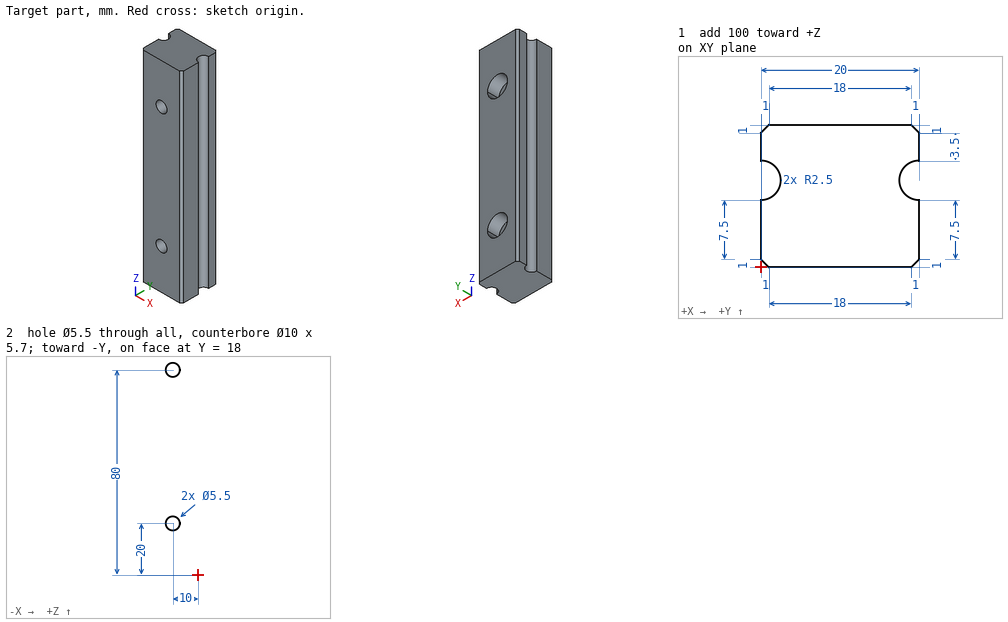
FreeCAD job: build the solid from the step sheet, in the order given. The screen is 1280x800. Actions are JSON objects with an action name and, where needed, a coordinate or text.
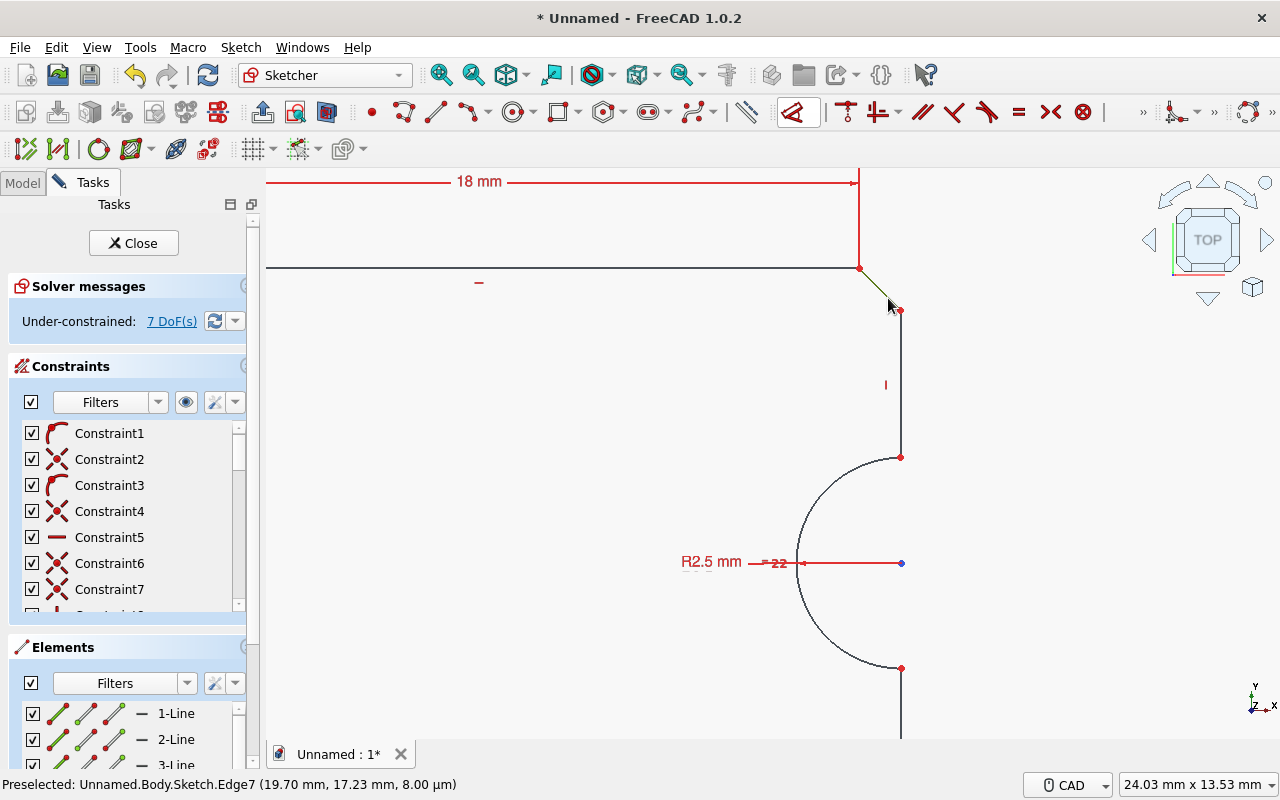
{"action": "key", "text": "l"}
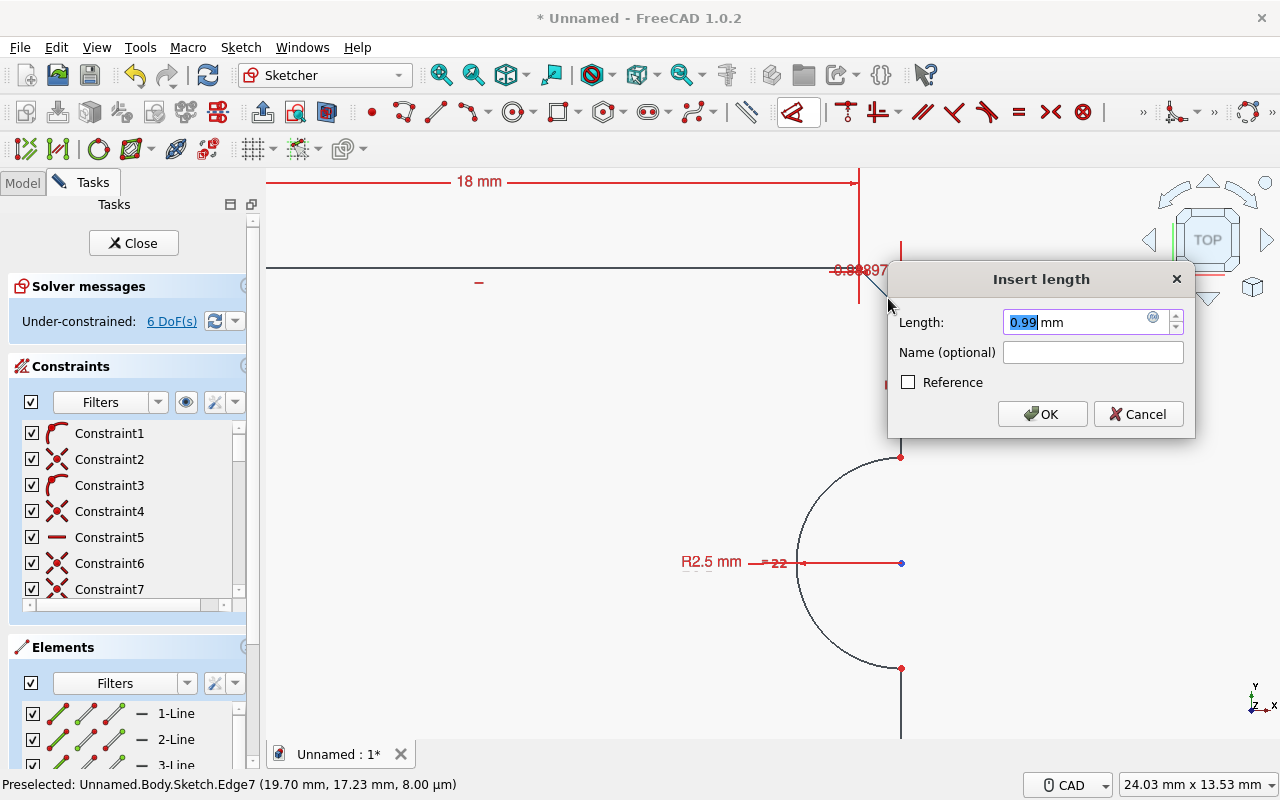
{"action": "type", "text": "1"}
{"action": "key", "text": "Return"}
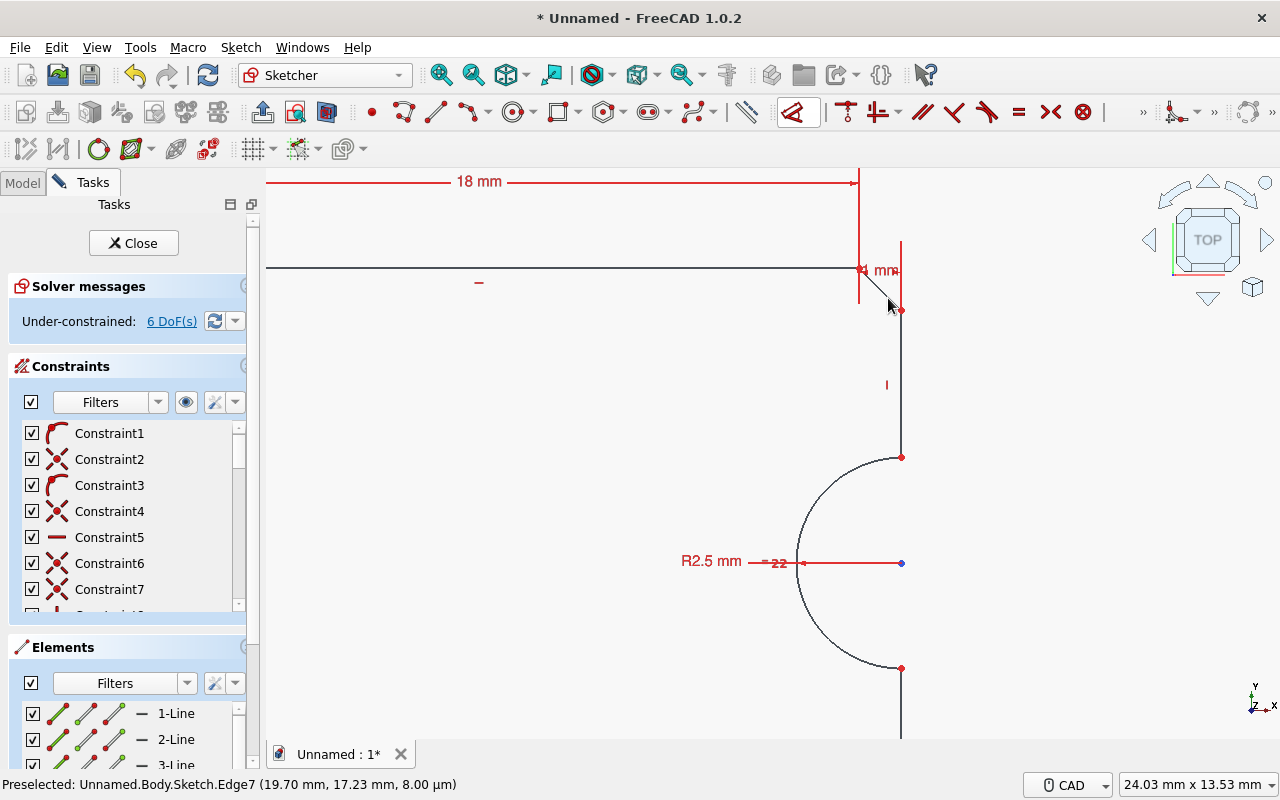
{"action": "left_click", "coordinate": [889, 298]}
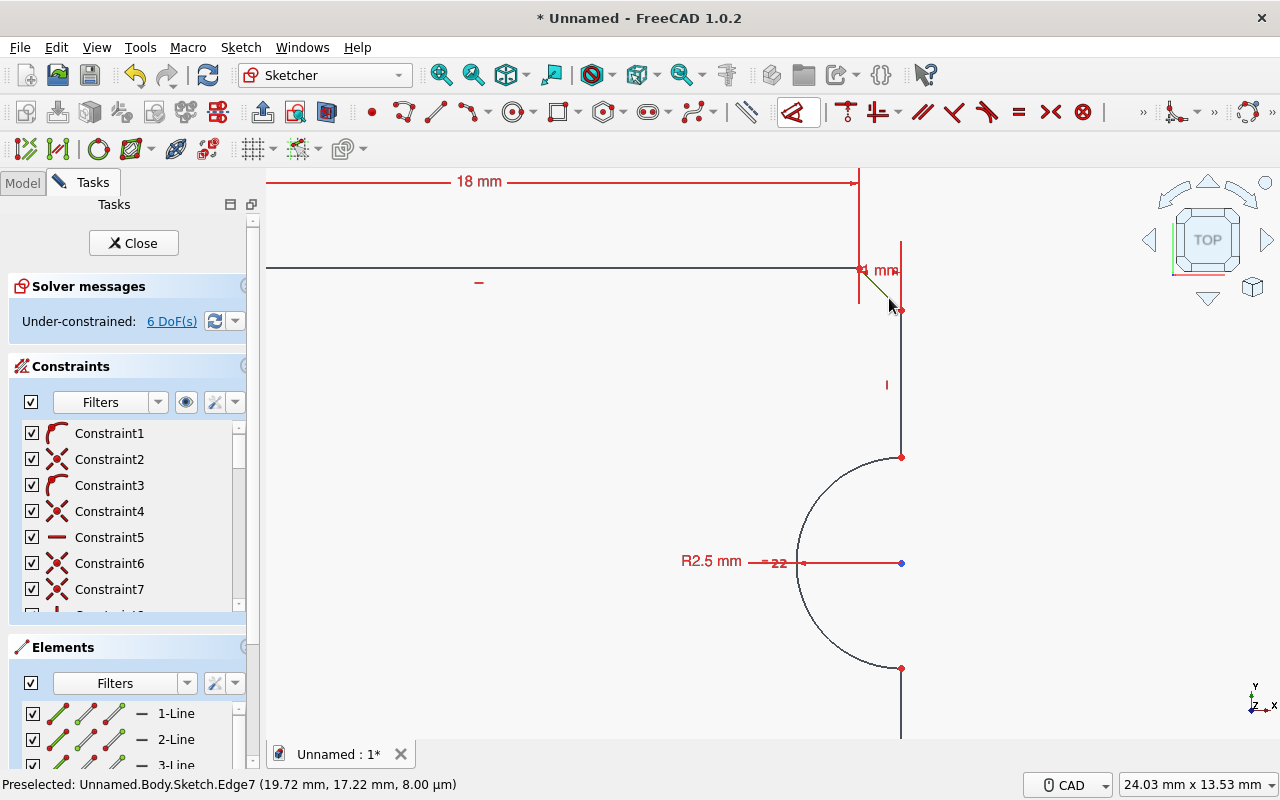
{"action": "left_click", "coordinate": [814, 112]}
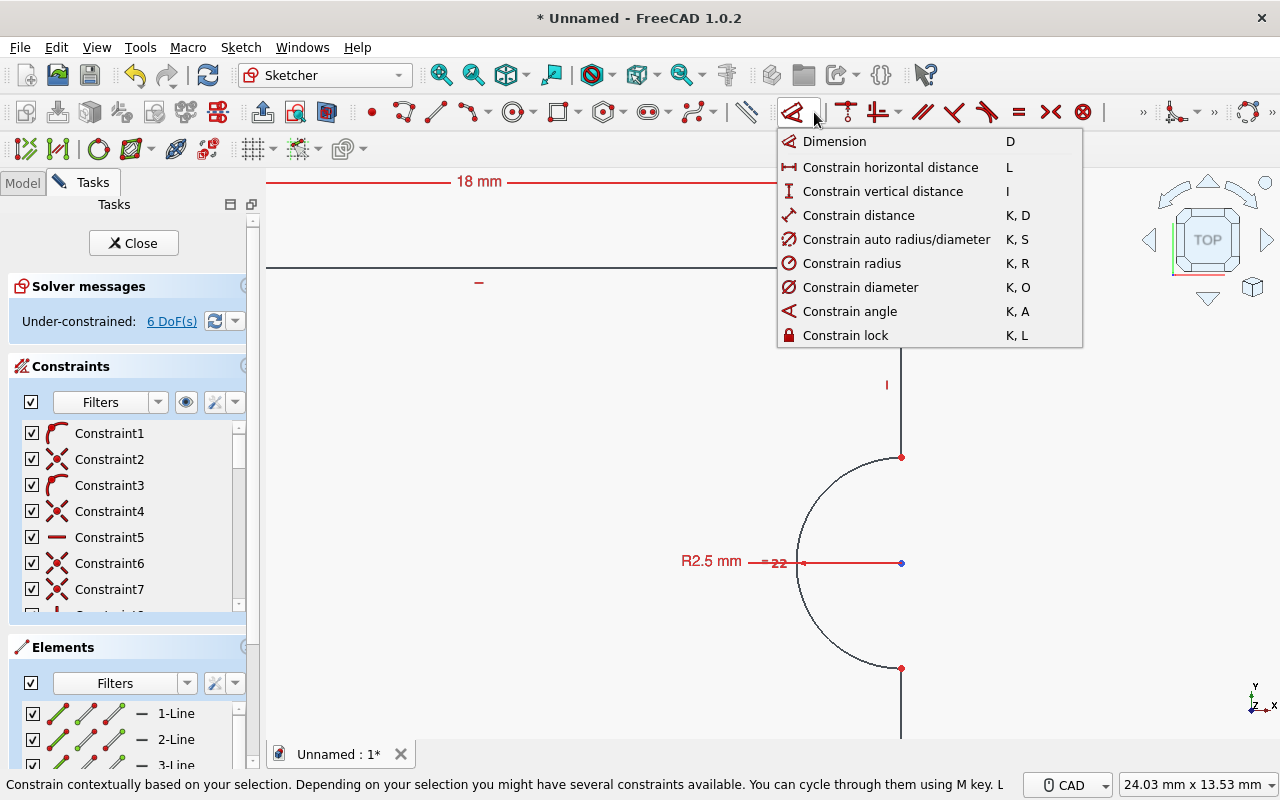
{"action": "left_click", "coordinate": [930, 191]}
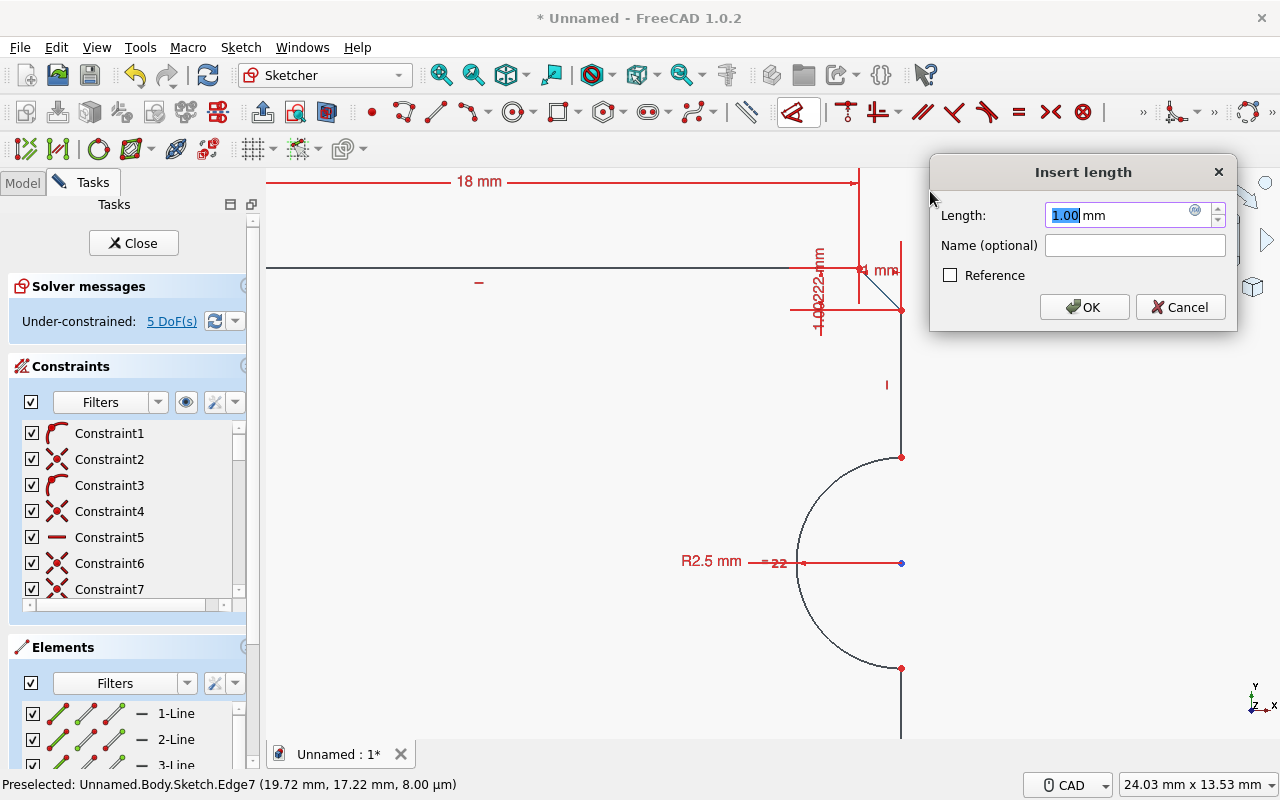
{"action": "type", "text": "1"}
{"action": "key", "text": "Return"}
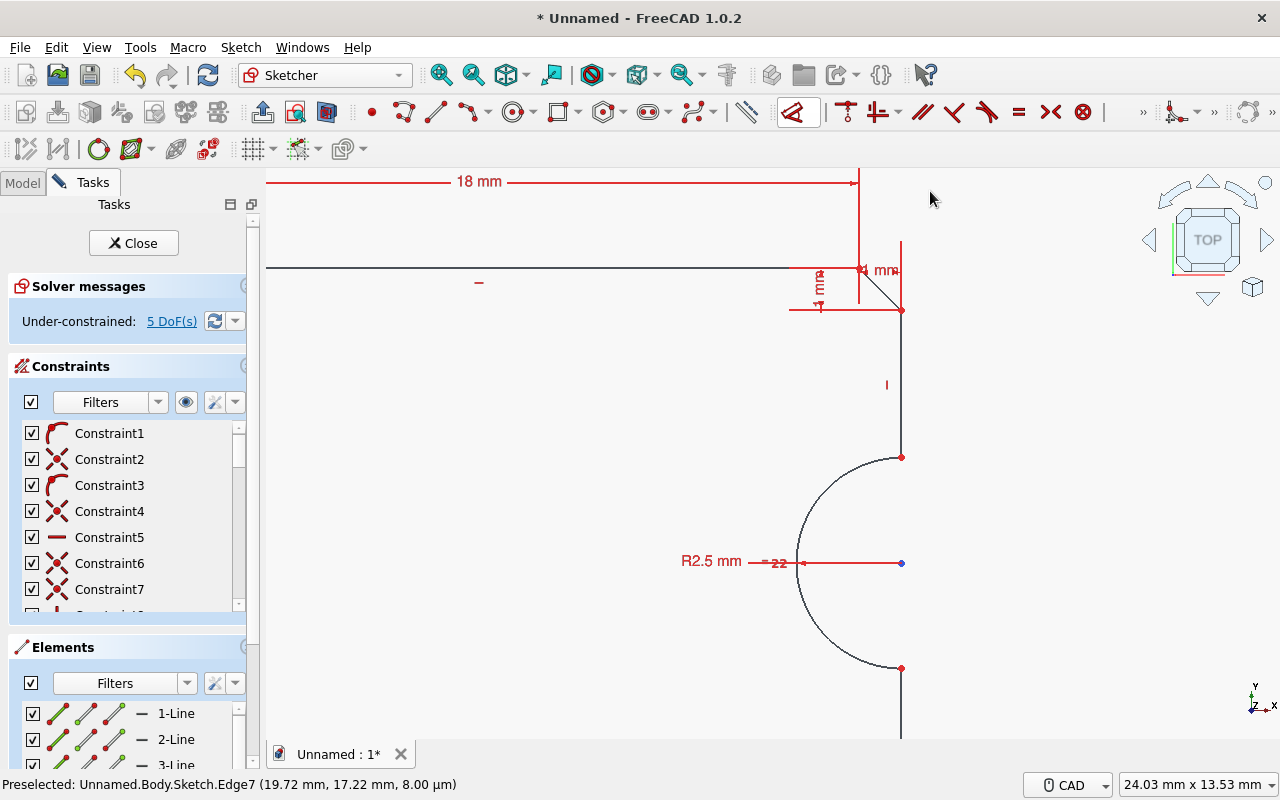
{"action": "scroll", "coordinate": [888, 297], "scroll_direction": "down", "scroll_amount": 4}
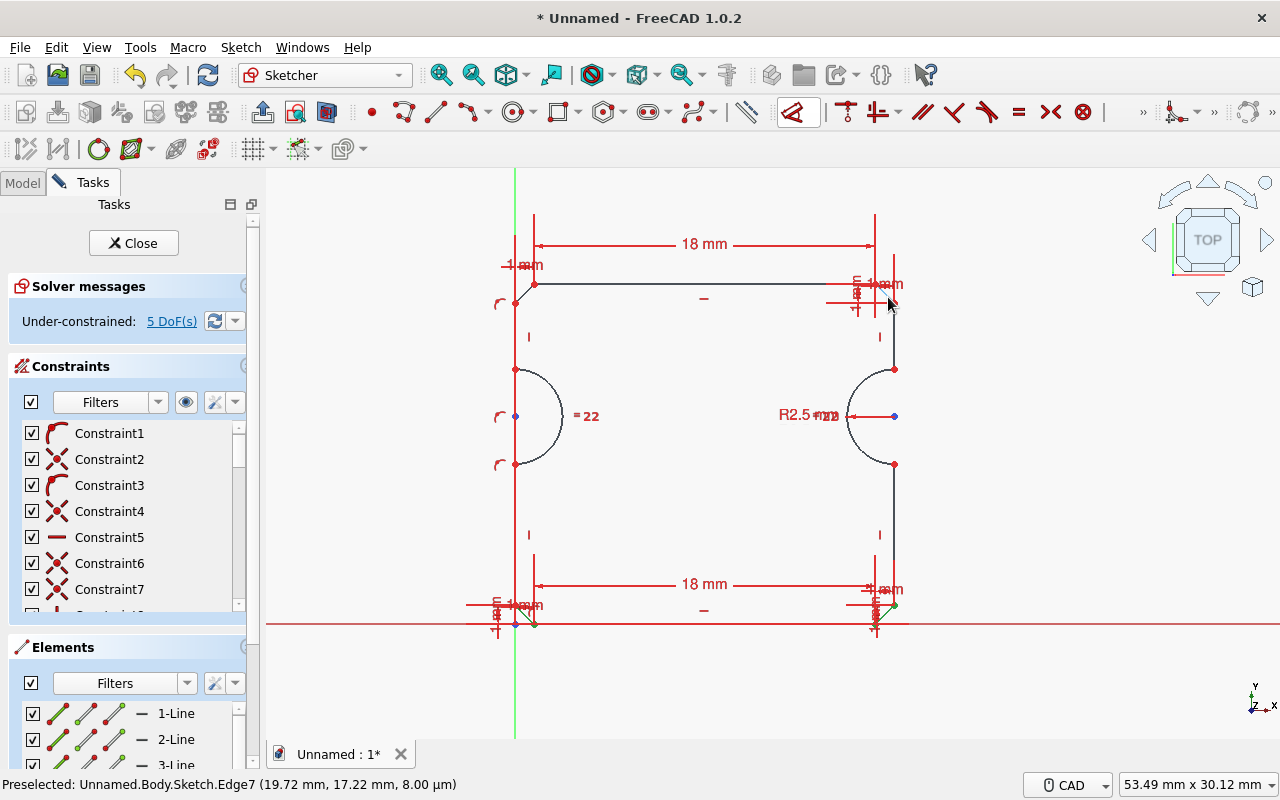
{"action": "scroll", "coordinate": [528, 290], "scroll_direction": "up", "scroll_amount": 4}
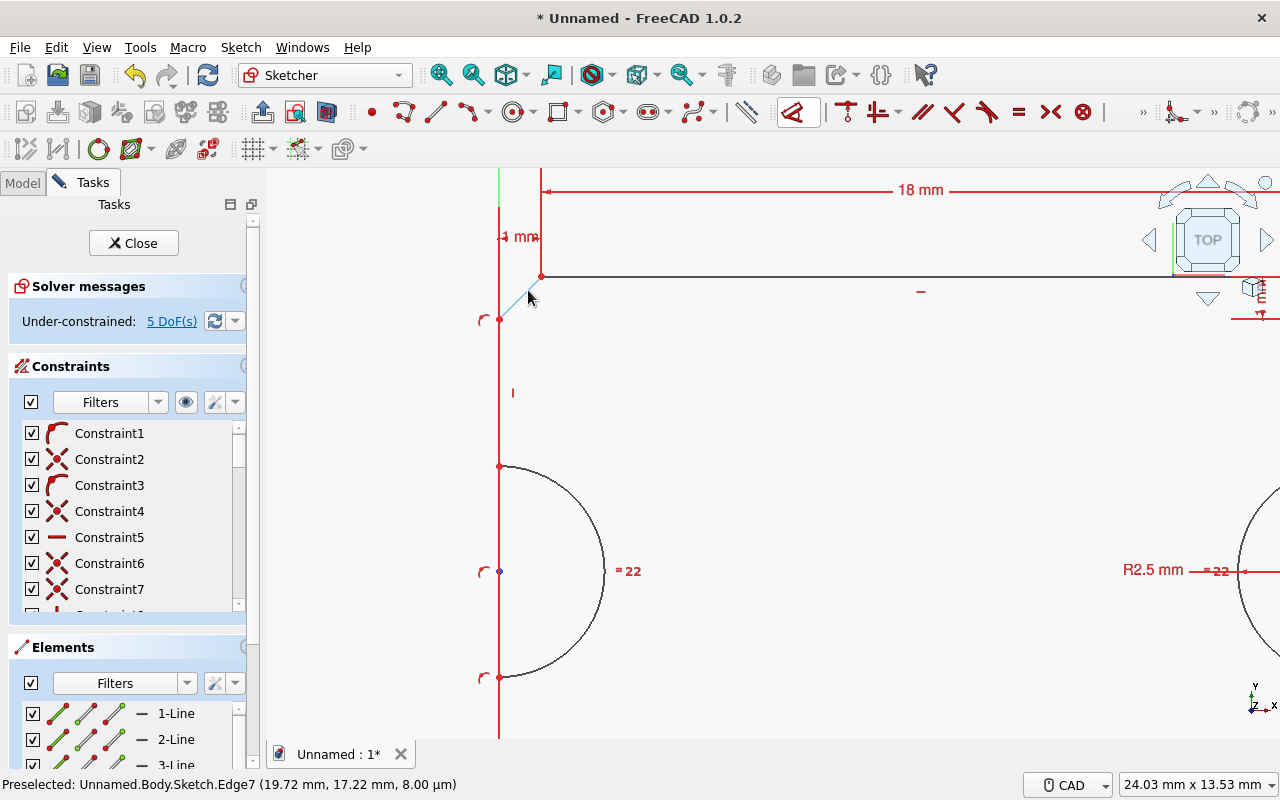
{"action": "left_click", "coordinate": [529, 289]}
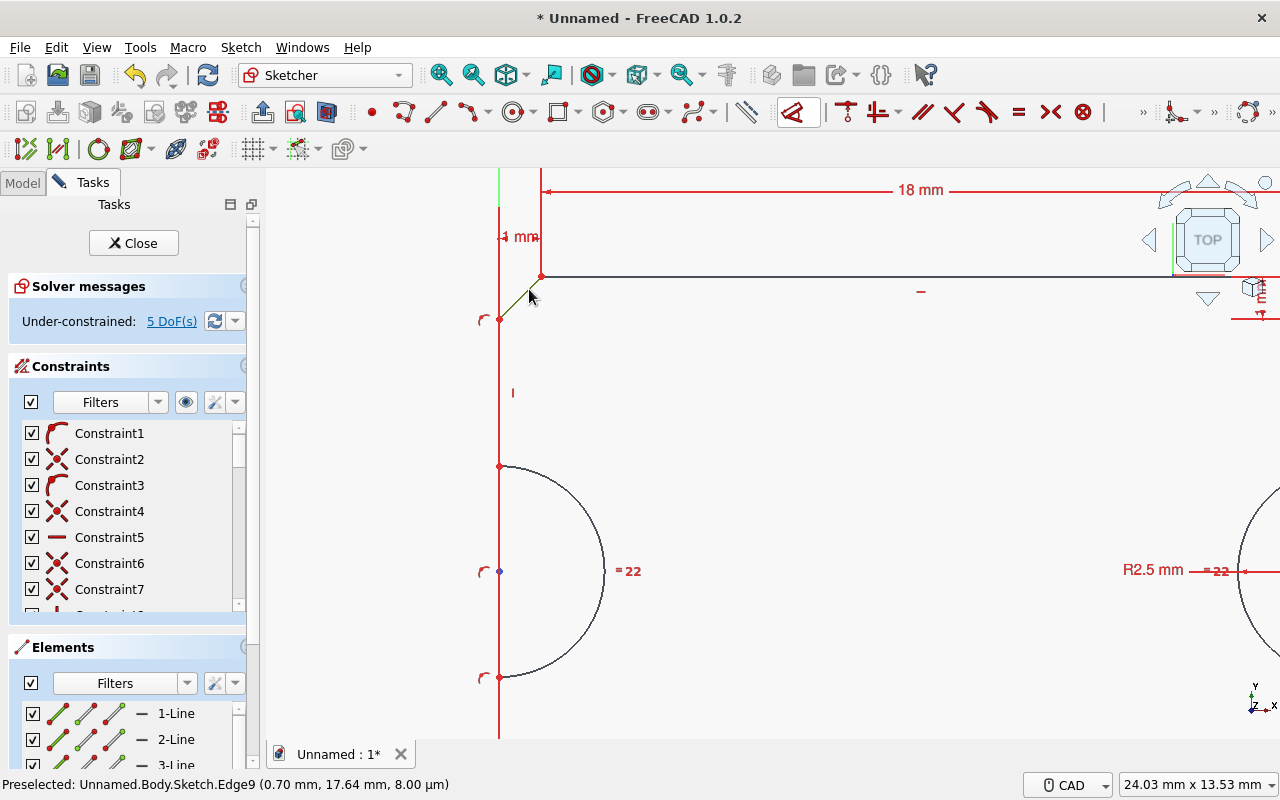
{"action": "key", "text": "i"}